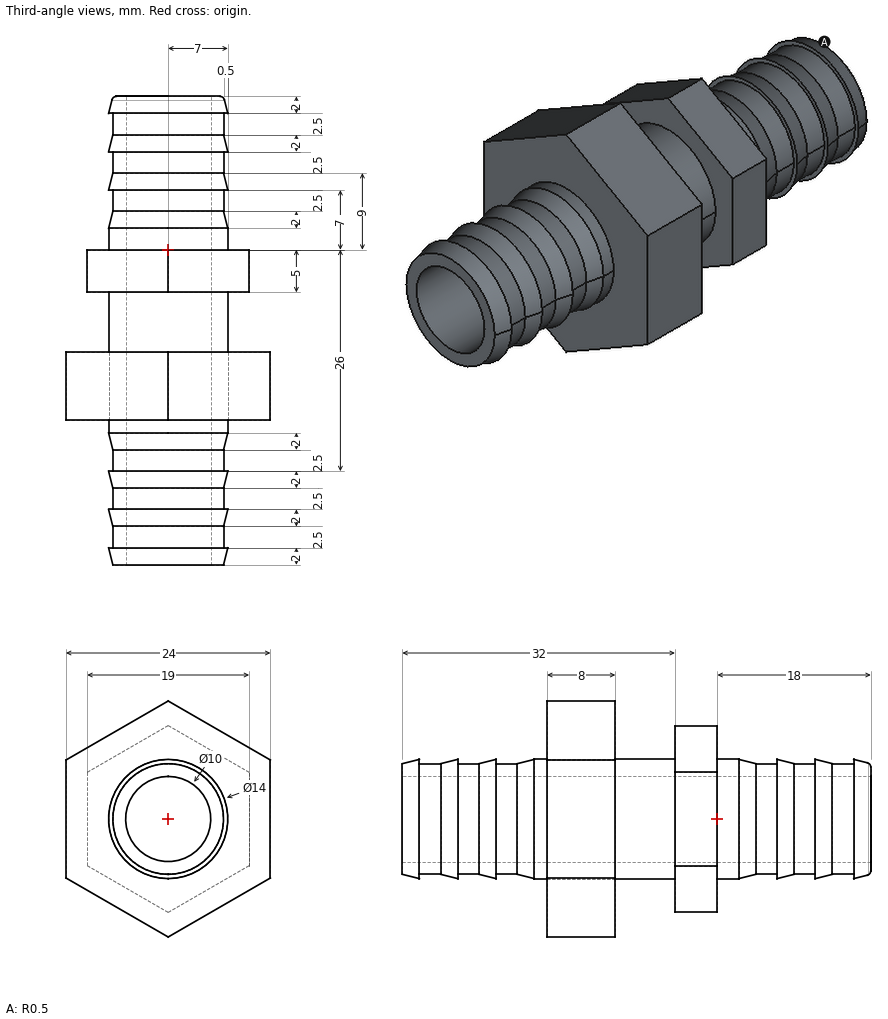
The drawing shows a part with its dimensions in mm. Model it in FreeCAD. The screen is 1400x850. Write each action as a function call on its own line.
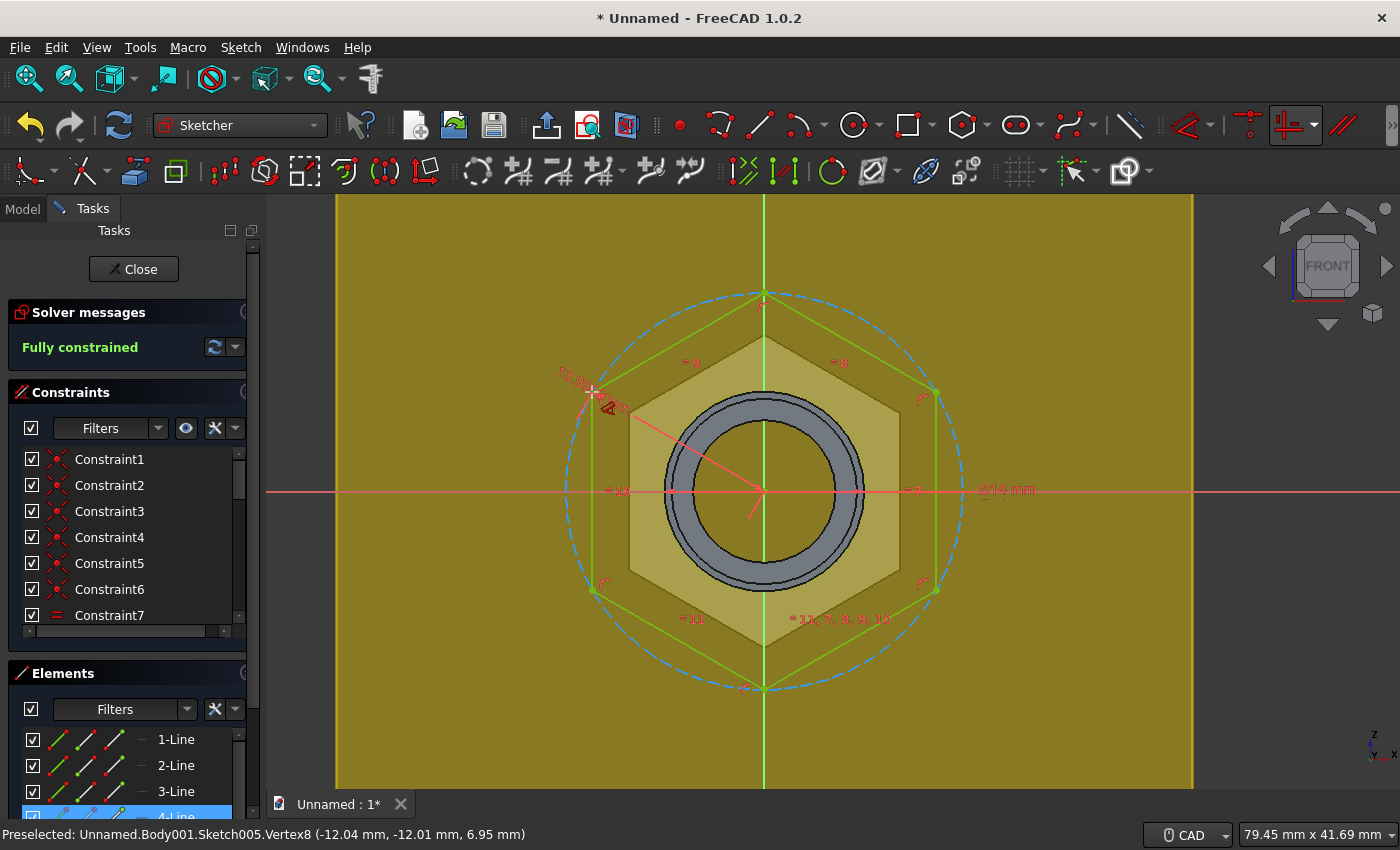
click(936, 591)
click(685, 358)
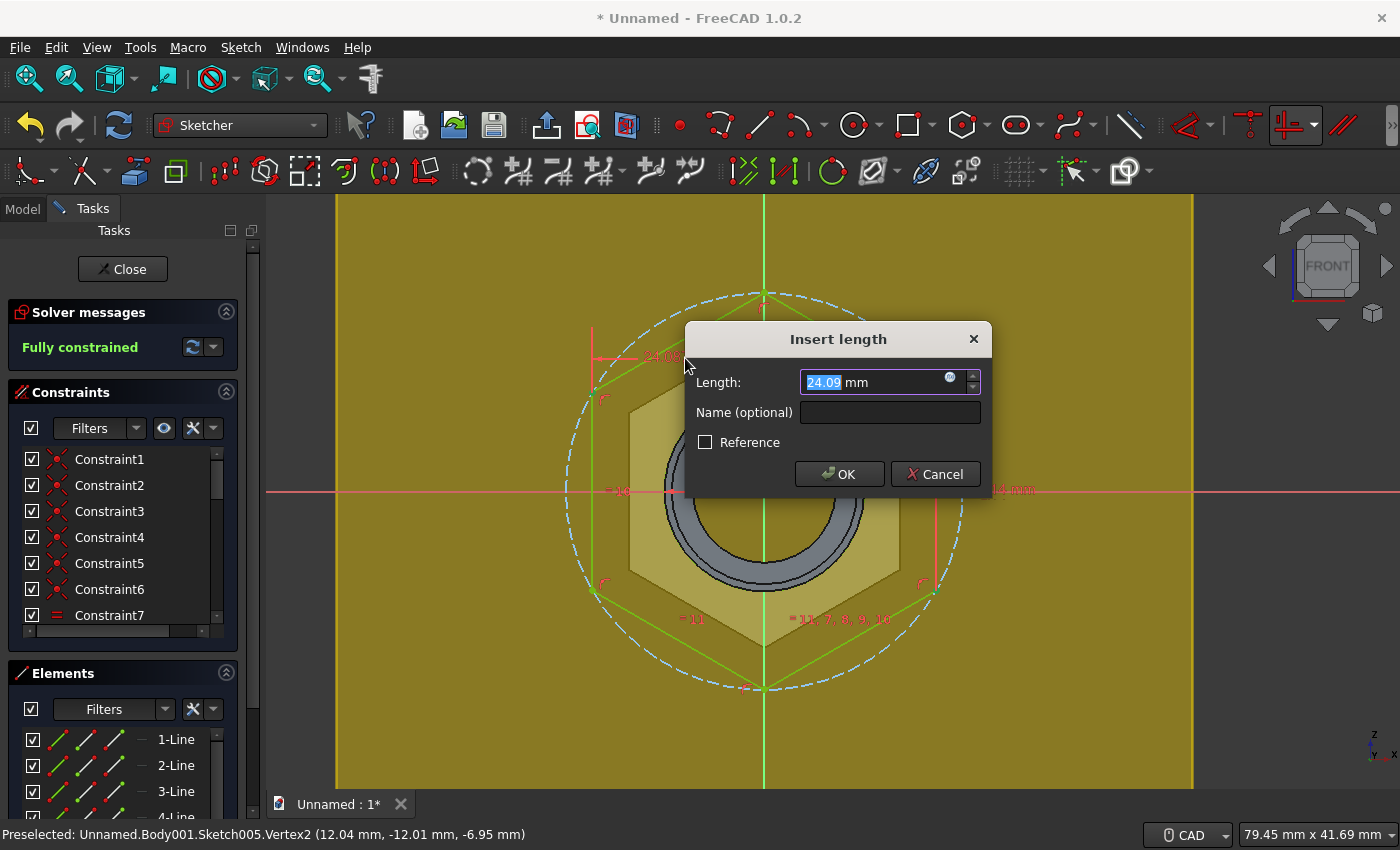
text(24)
key(Return)
key(Escape)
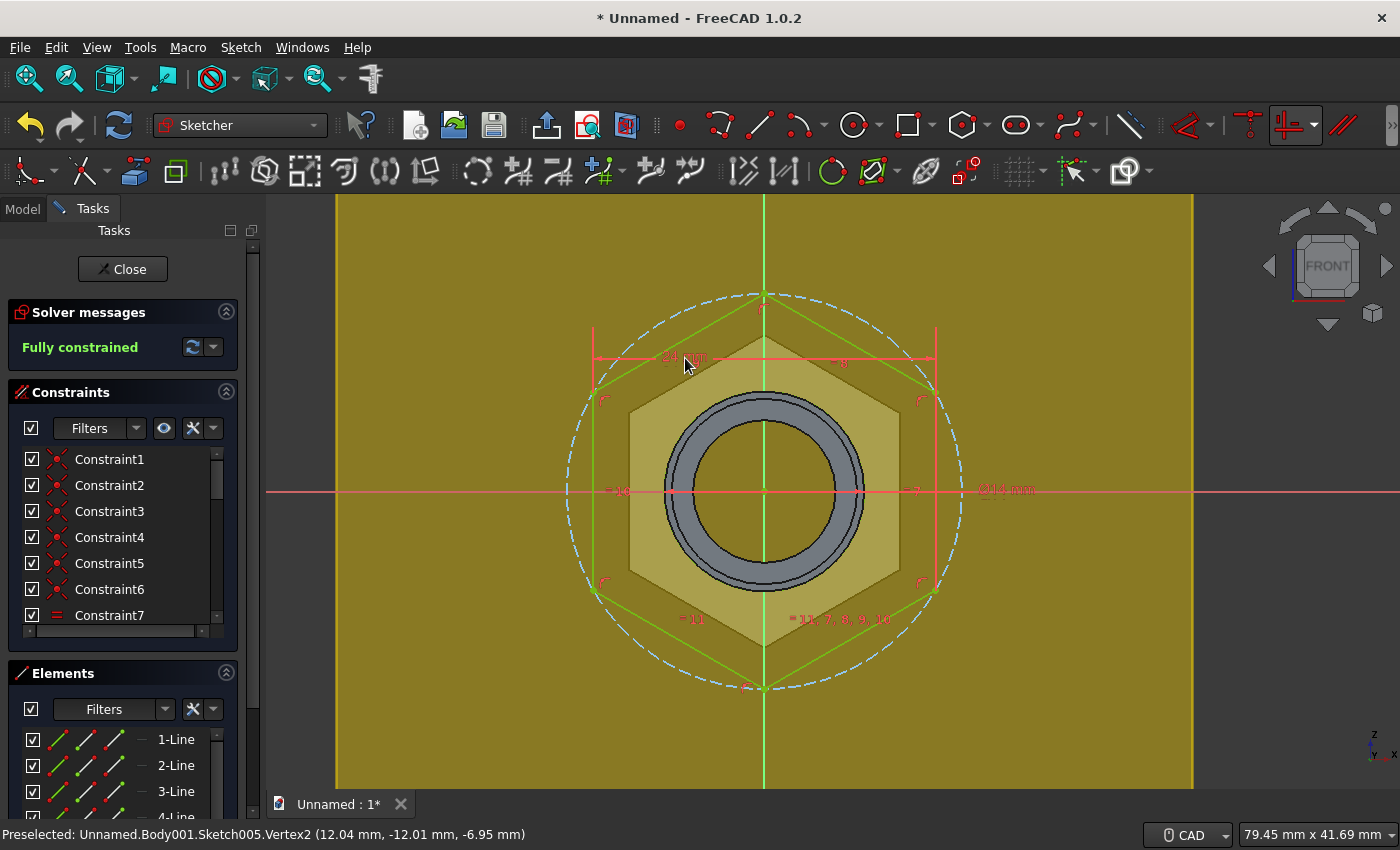
click(123, 269)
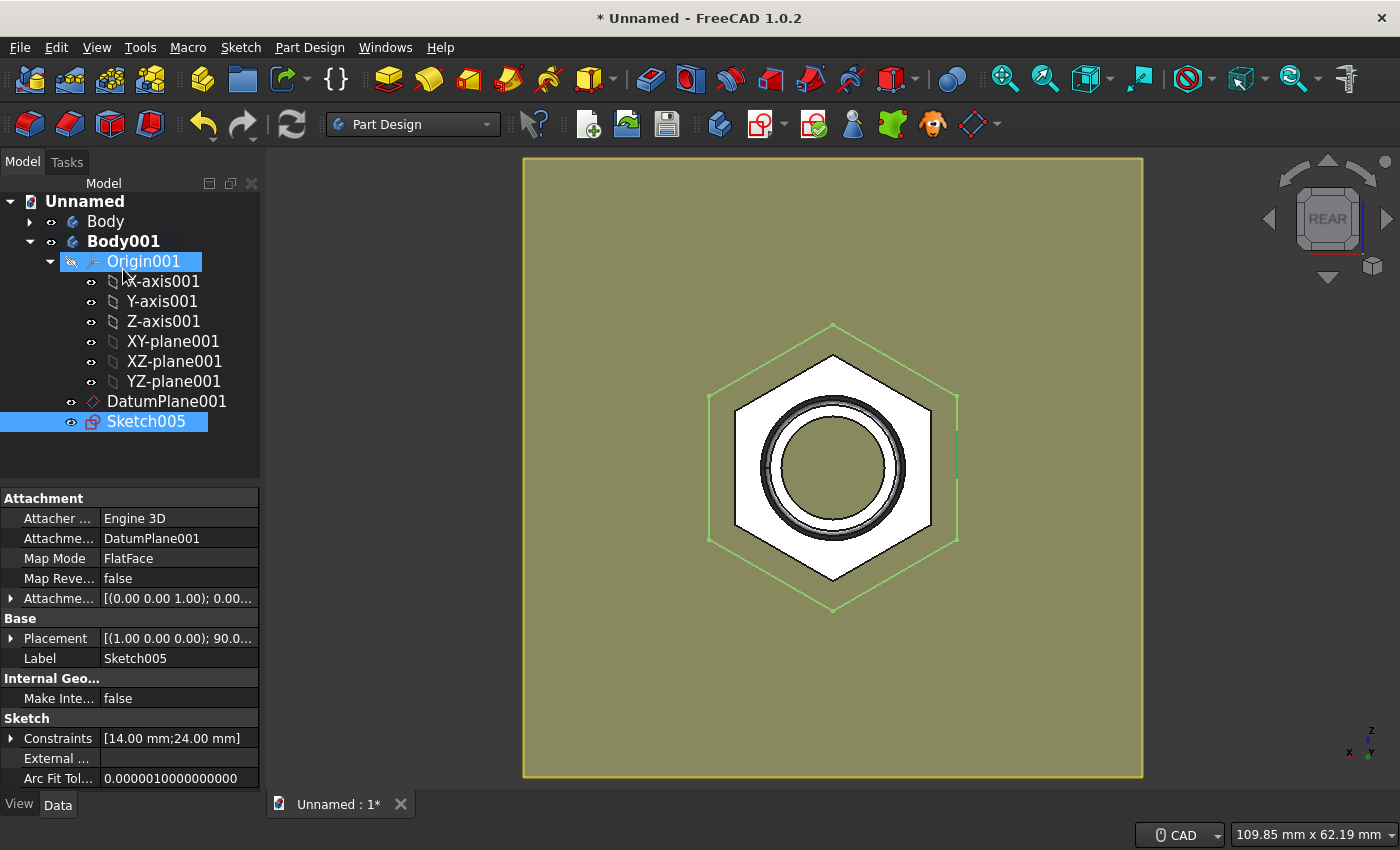
click(390, 80)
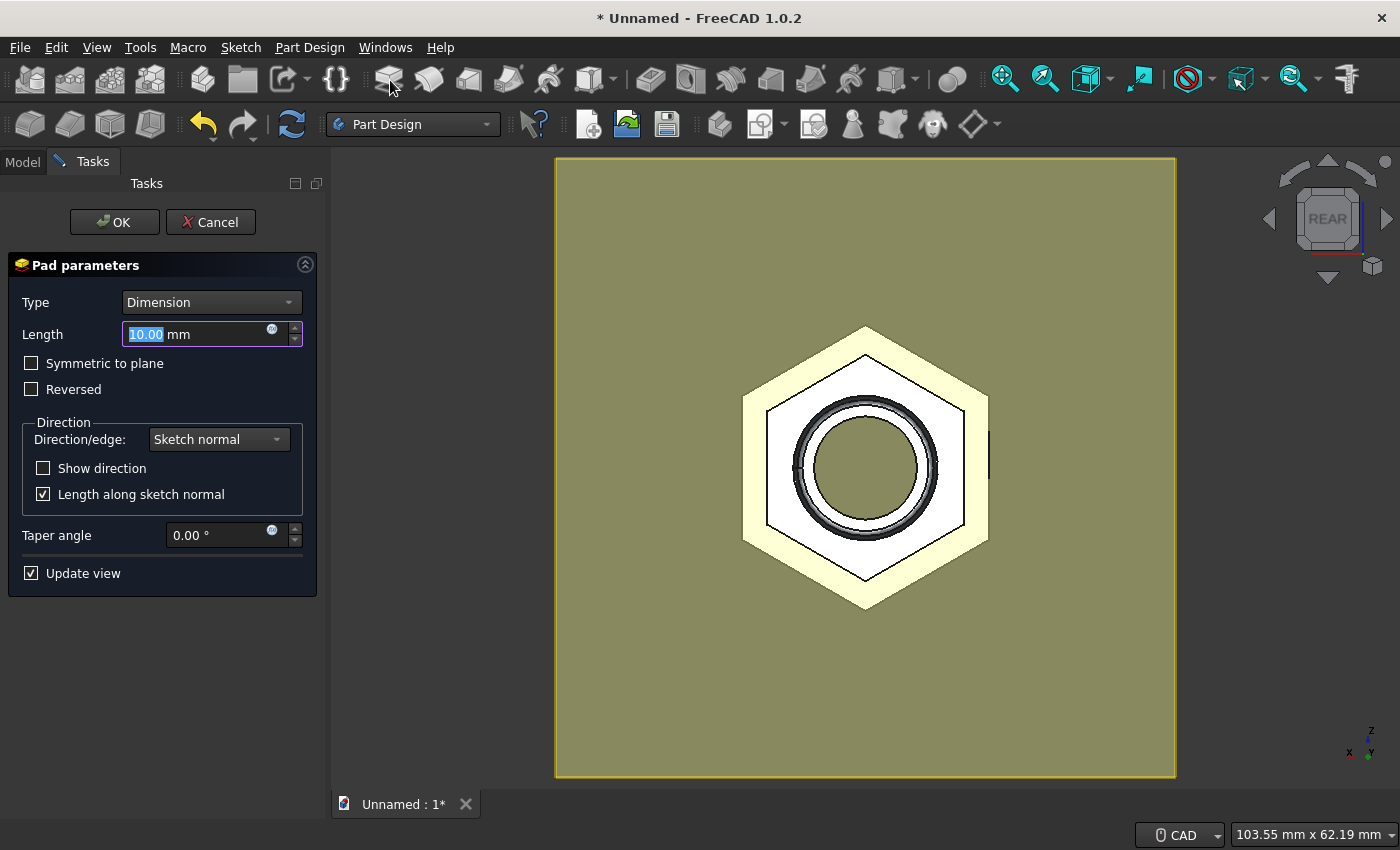
text(8)
key(Tab)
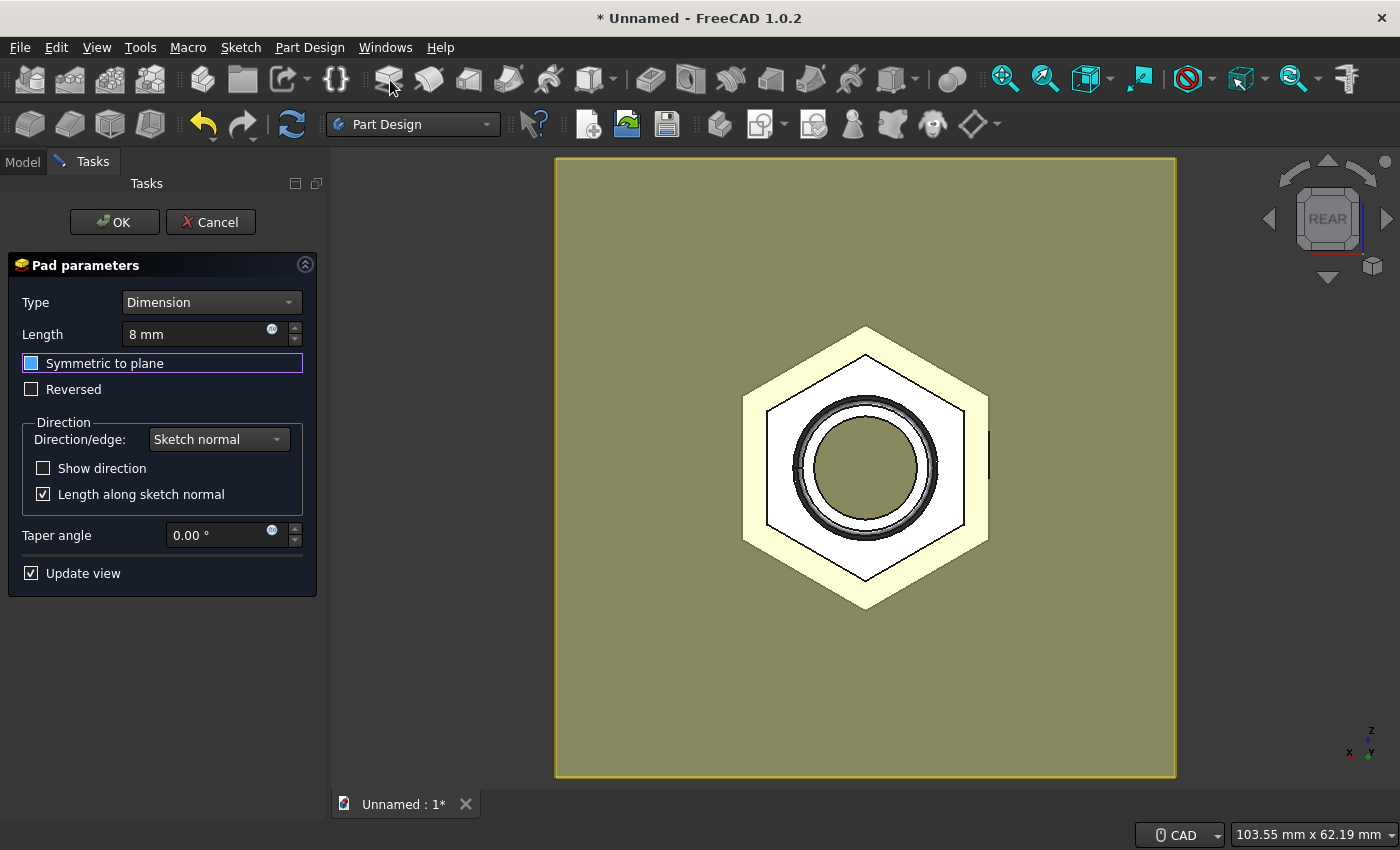
click(115, 222)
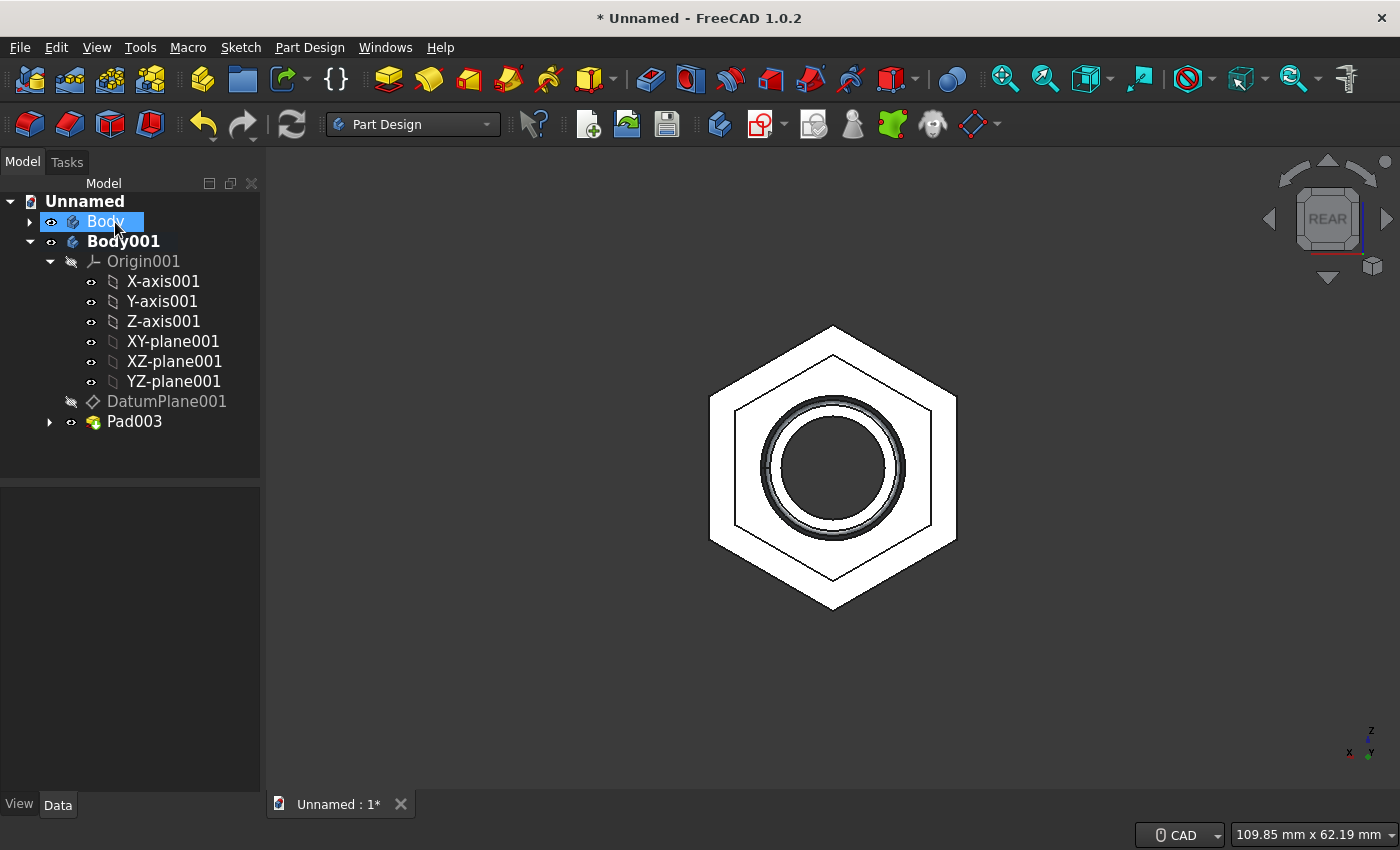
key(0)